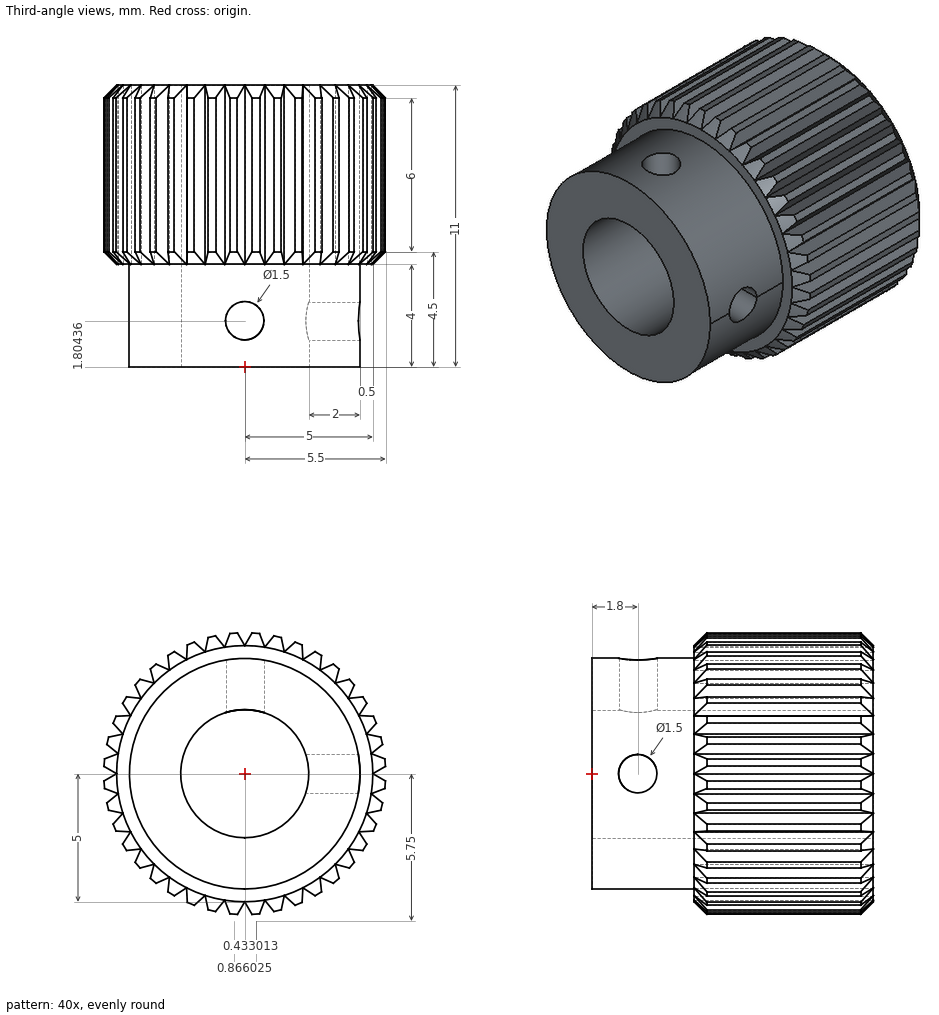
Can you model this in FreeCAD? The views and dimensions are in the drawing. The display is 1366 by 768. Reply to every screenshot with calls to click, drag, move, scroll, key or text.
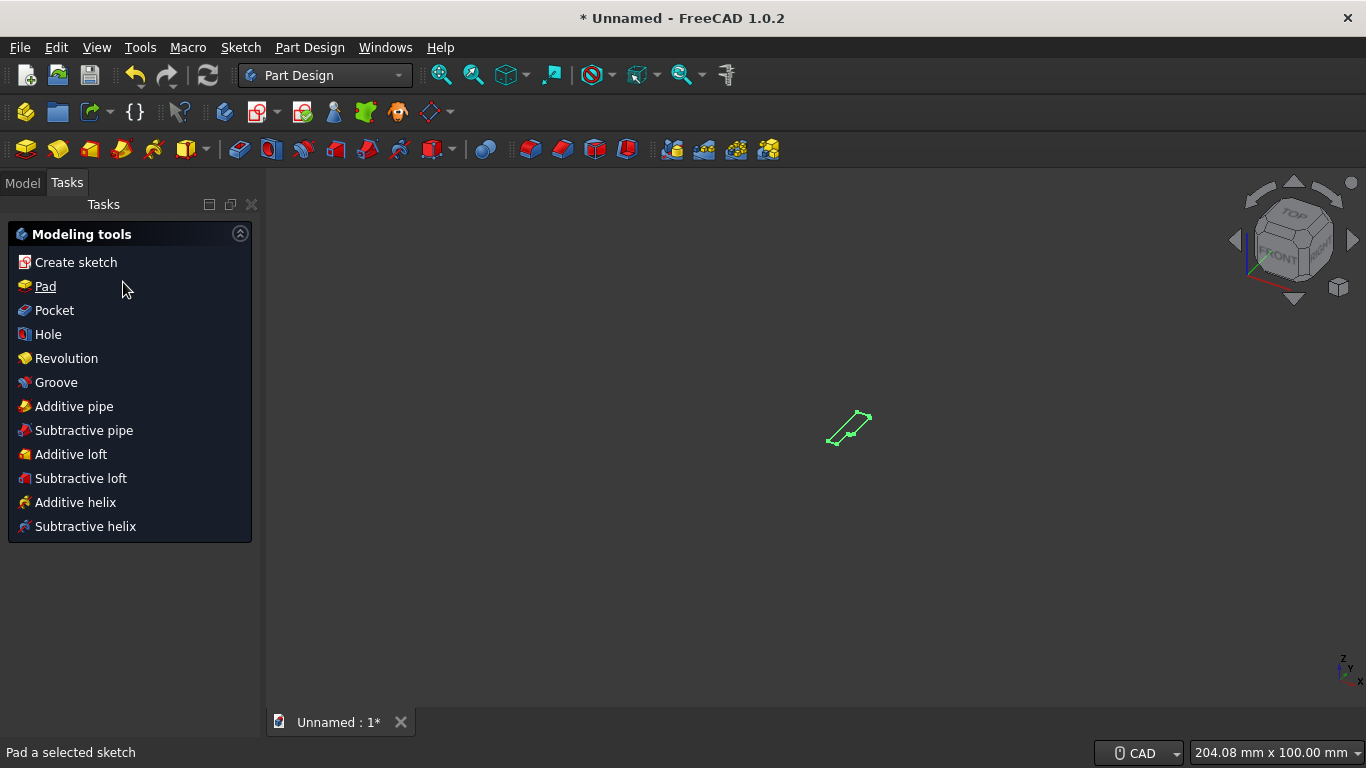
click(58, 150)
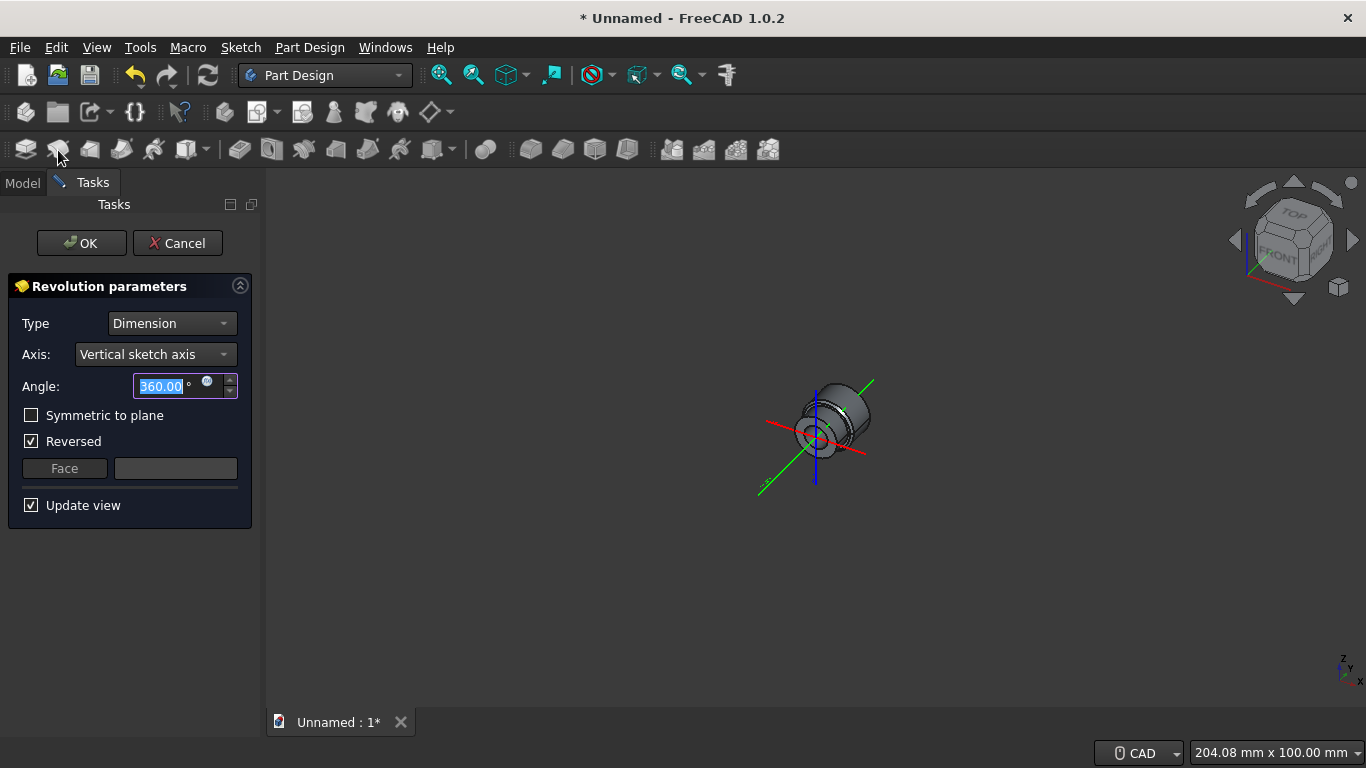
click(82, 243)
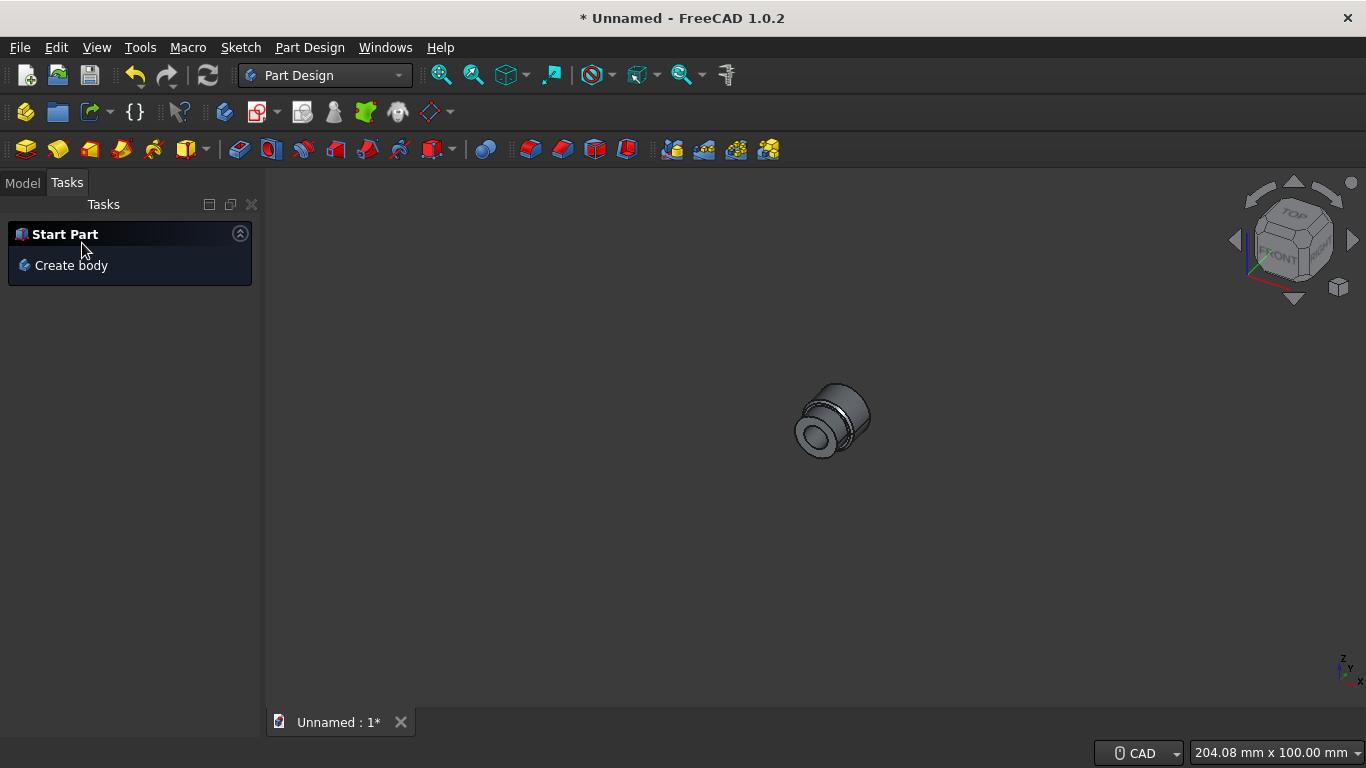
key(v)
key(f)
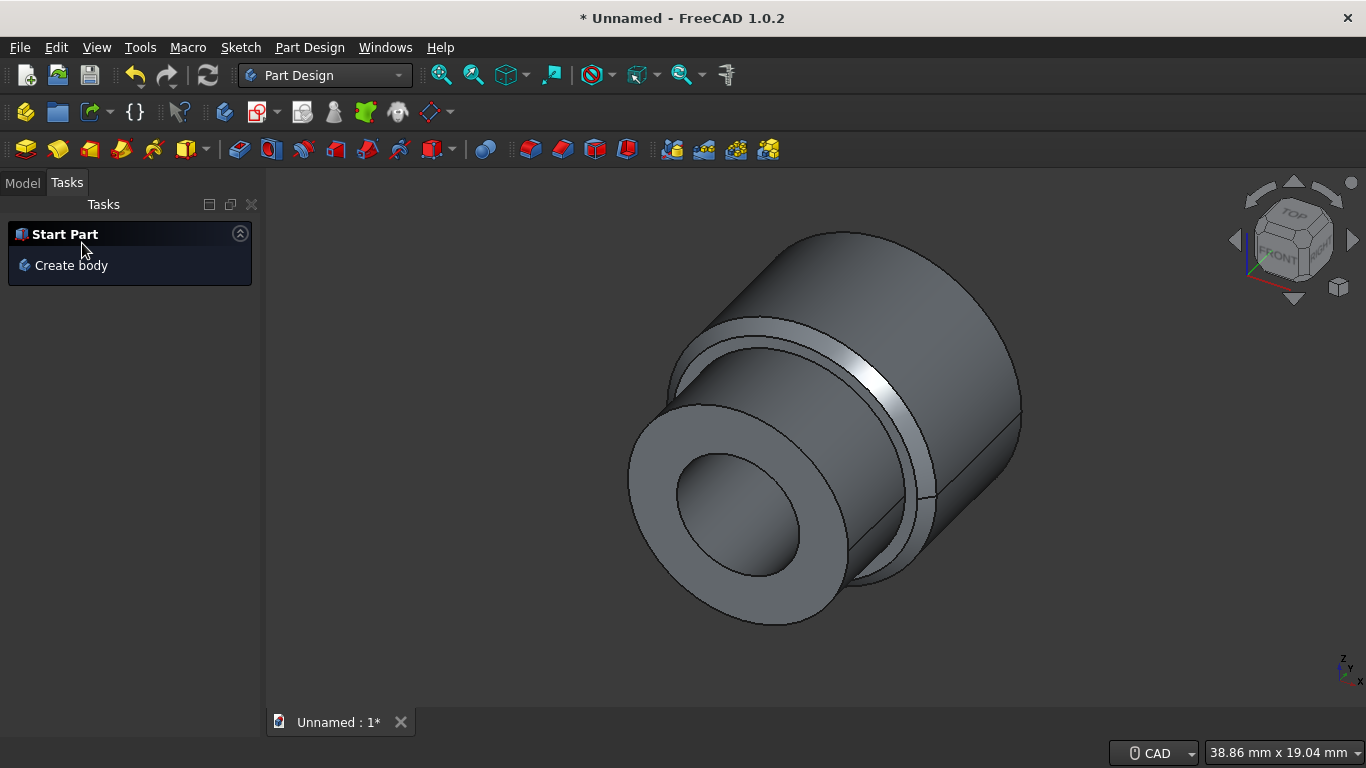
key(4)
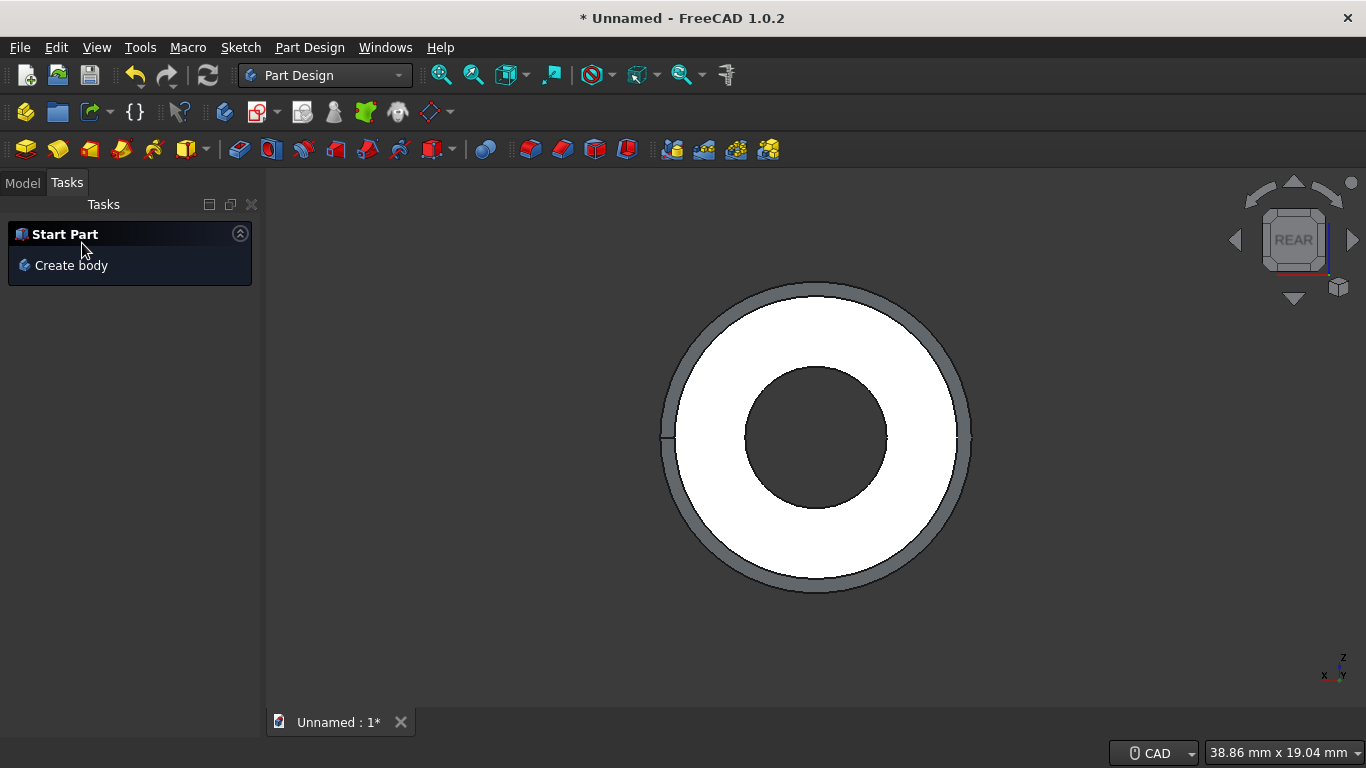
click(735, 356)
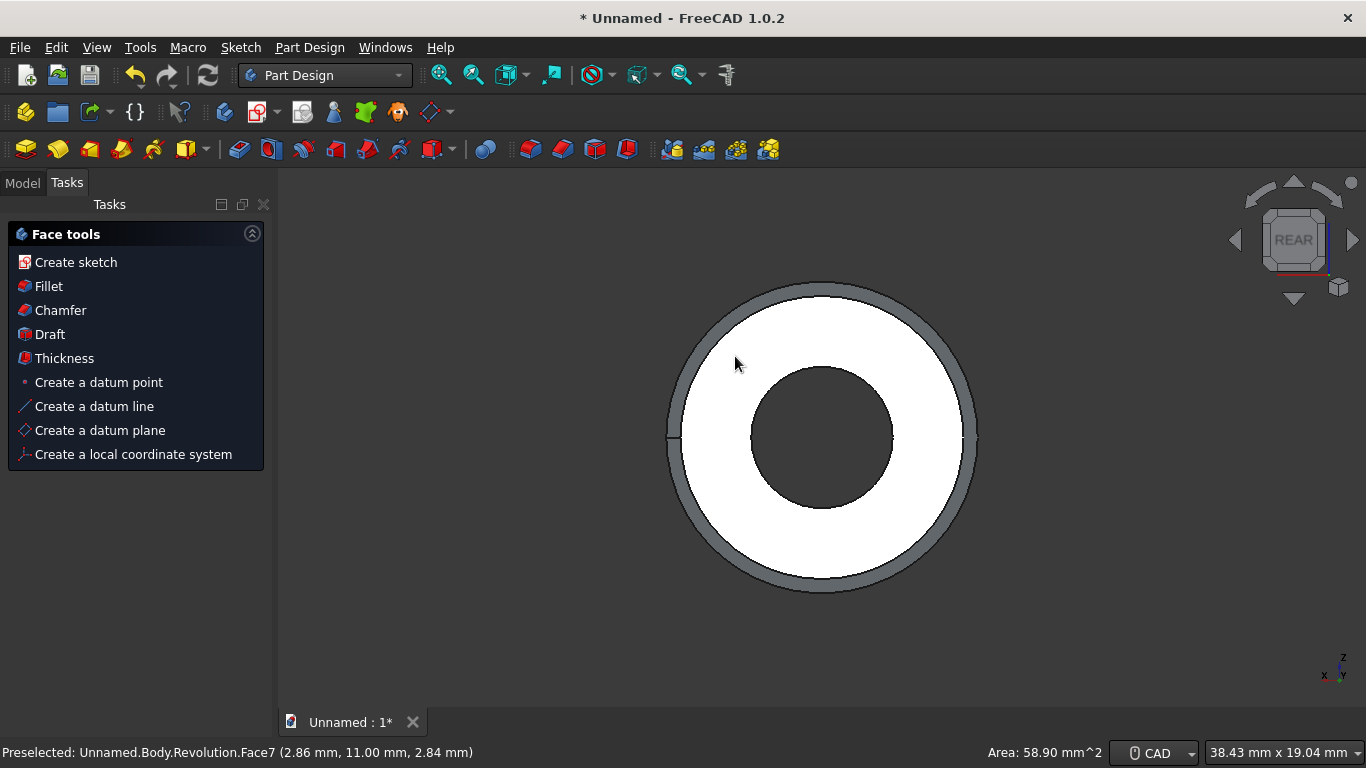
click(258, 112)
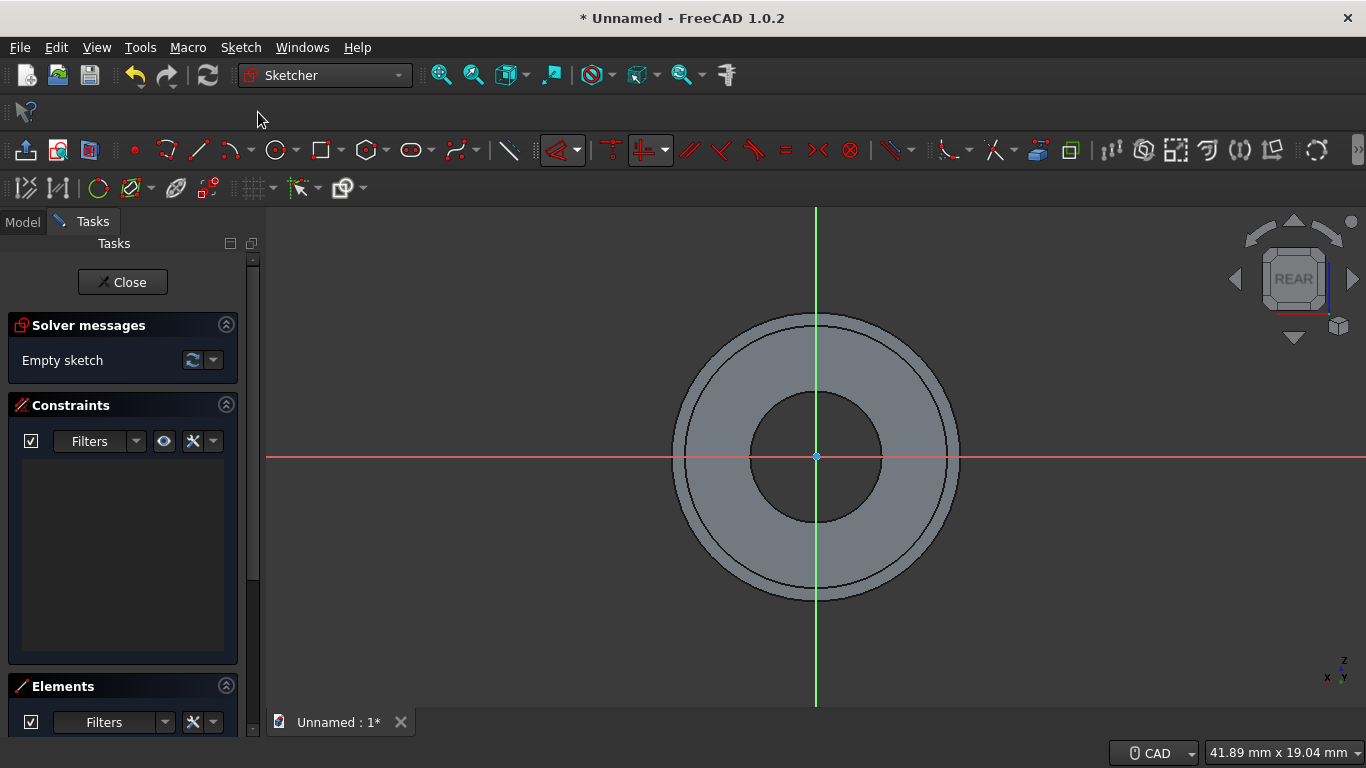
scroll(820, 607, up, 14)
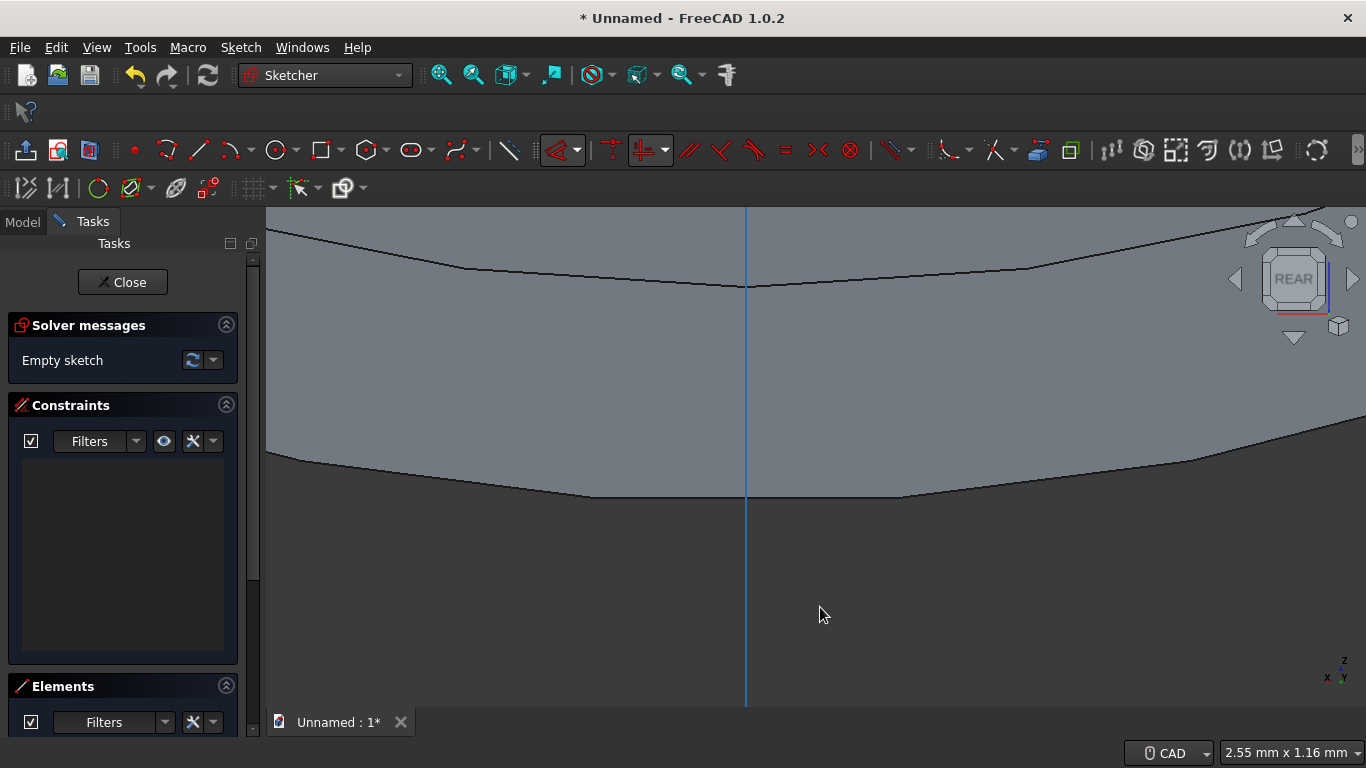
key(g)
key(m)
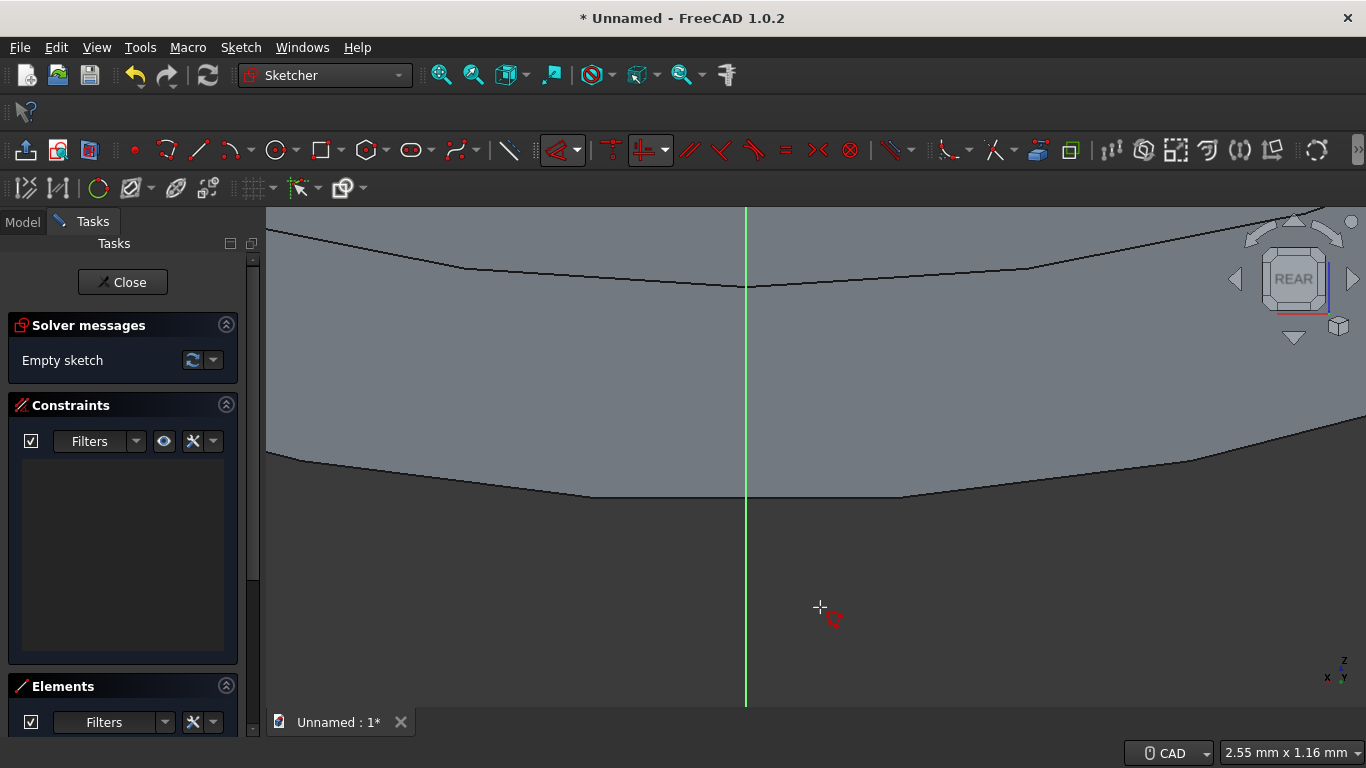
click(746, 287)
click(559, 611)
click(933, 611)
click(746, 288)
key(Escape)
key(Escape)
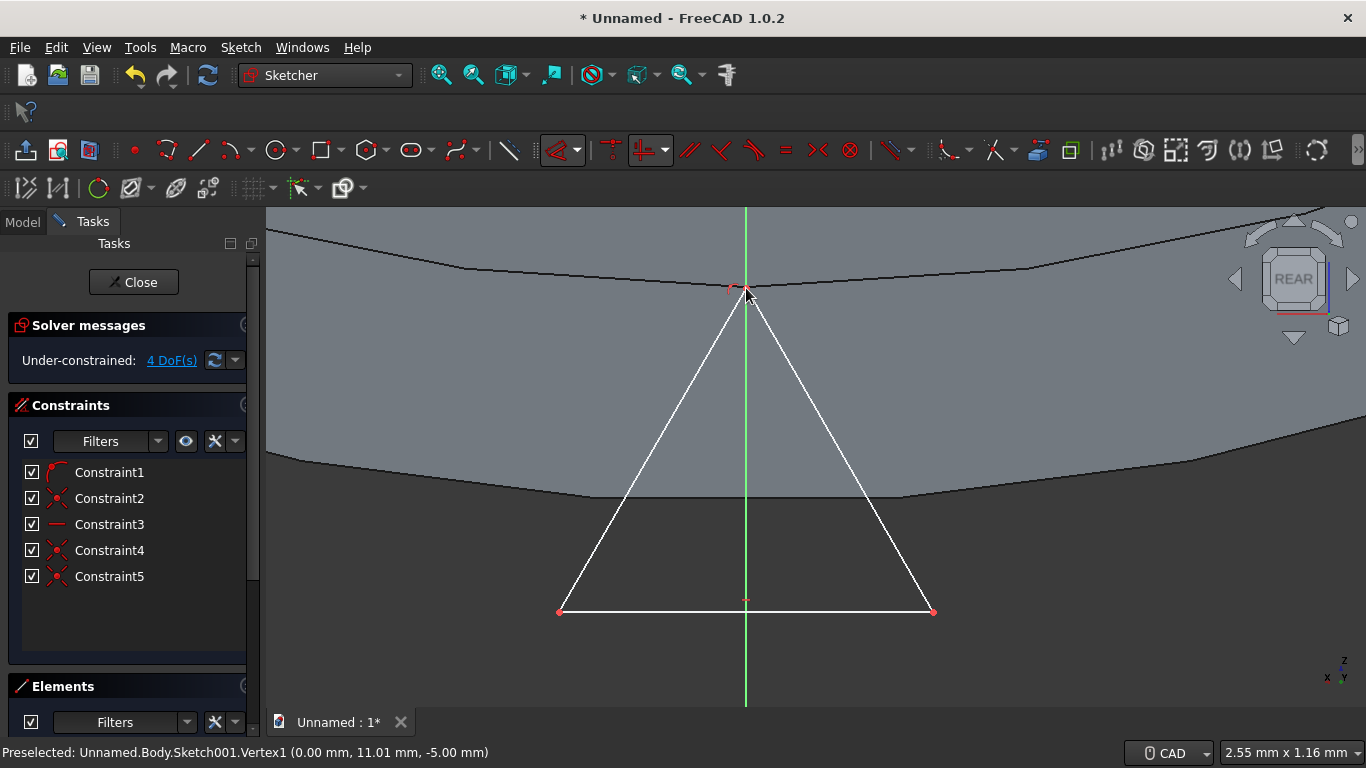
click(746, 288)